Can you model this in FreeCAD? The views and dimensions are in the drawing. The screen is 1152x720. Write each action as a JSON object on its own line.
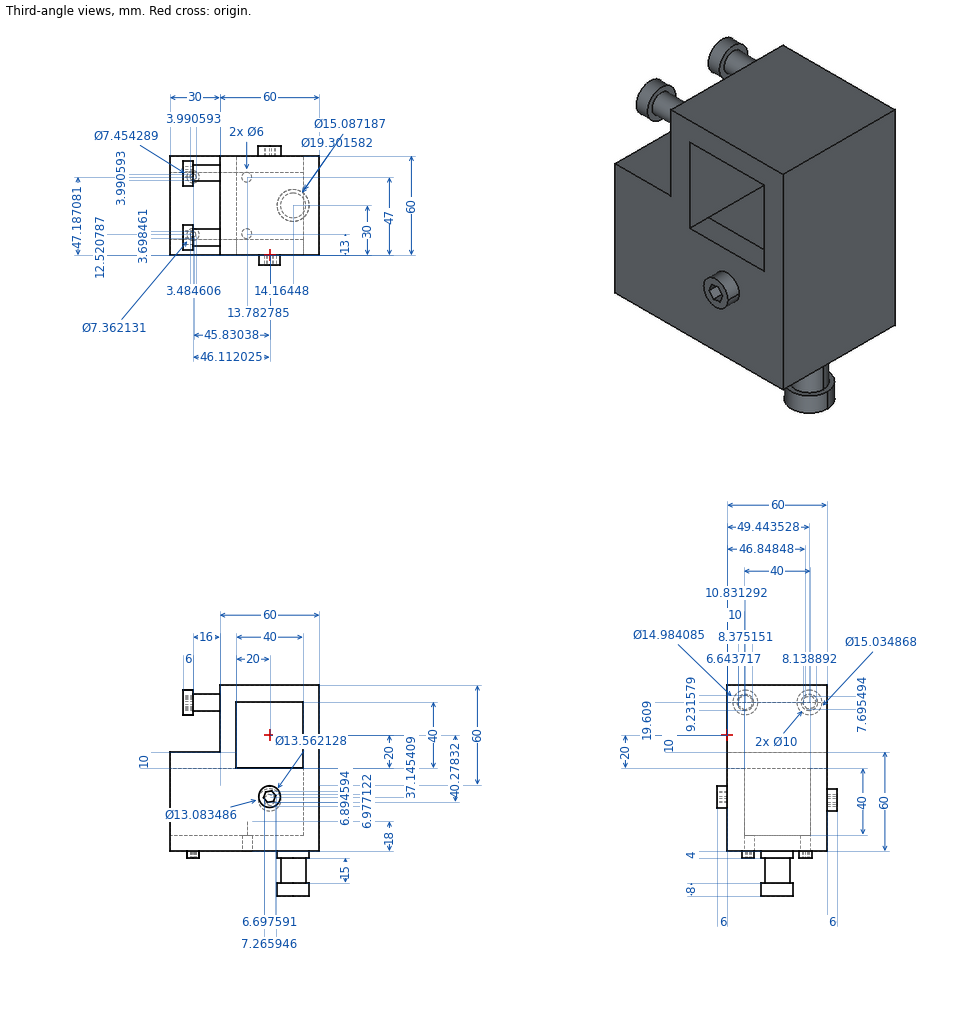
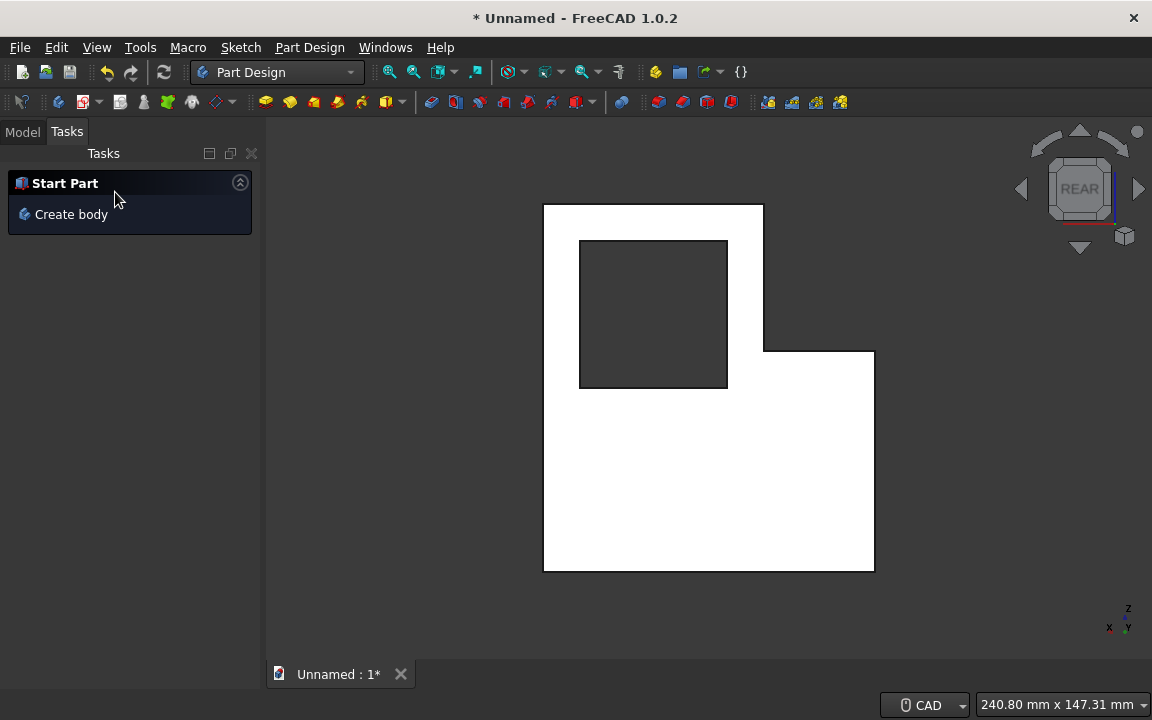
{"action": "key", "text": "5"}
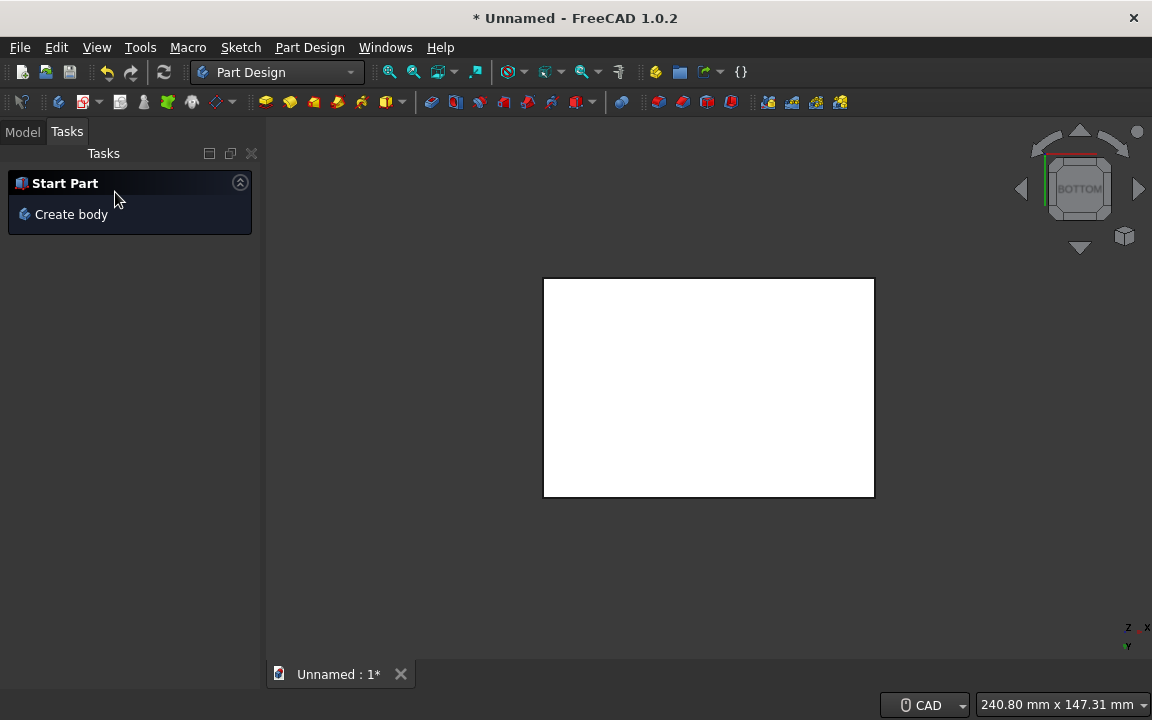
{"action": "left_click", "coordinate": [390, 72]}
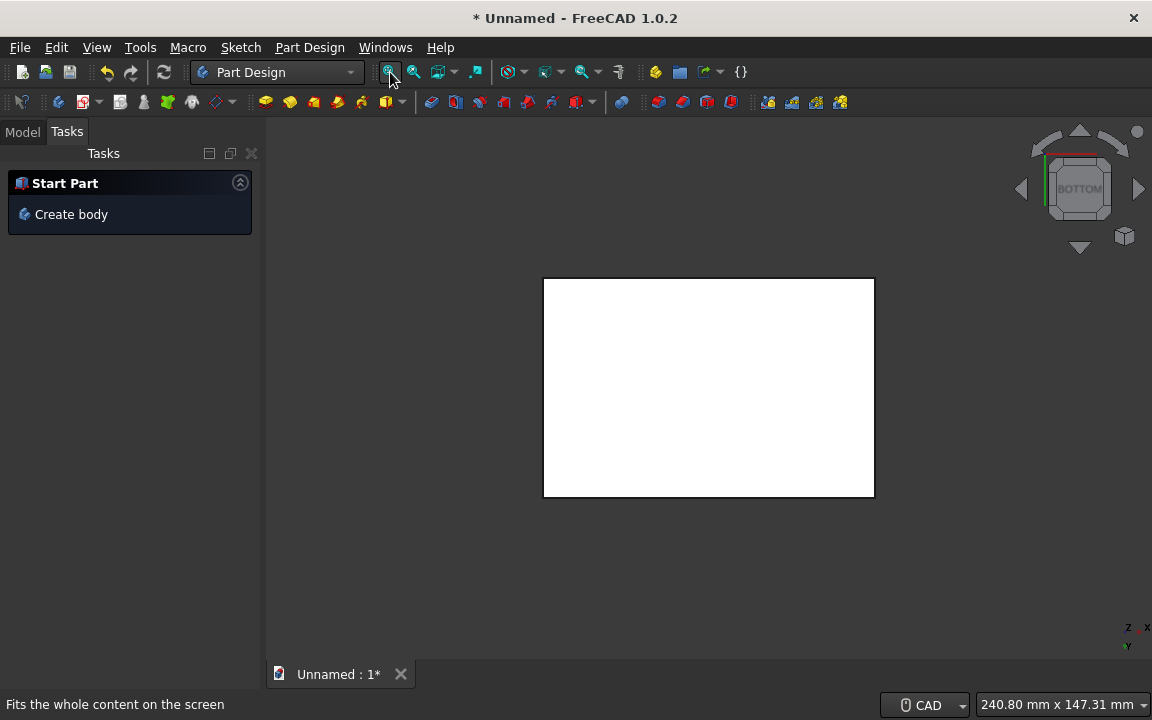
{"action": "left_click", "coordinate": [756, 387]}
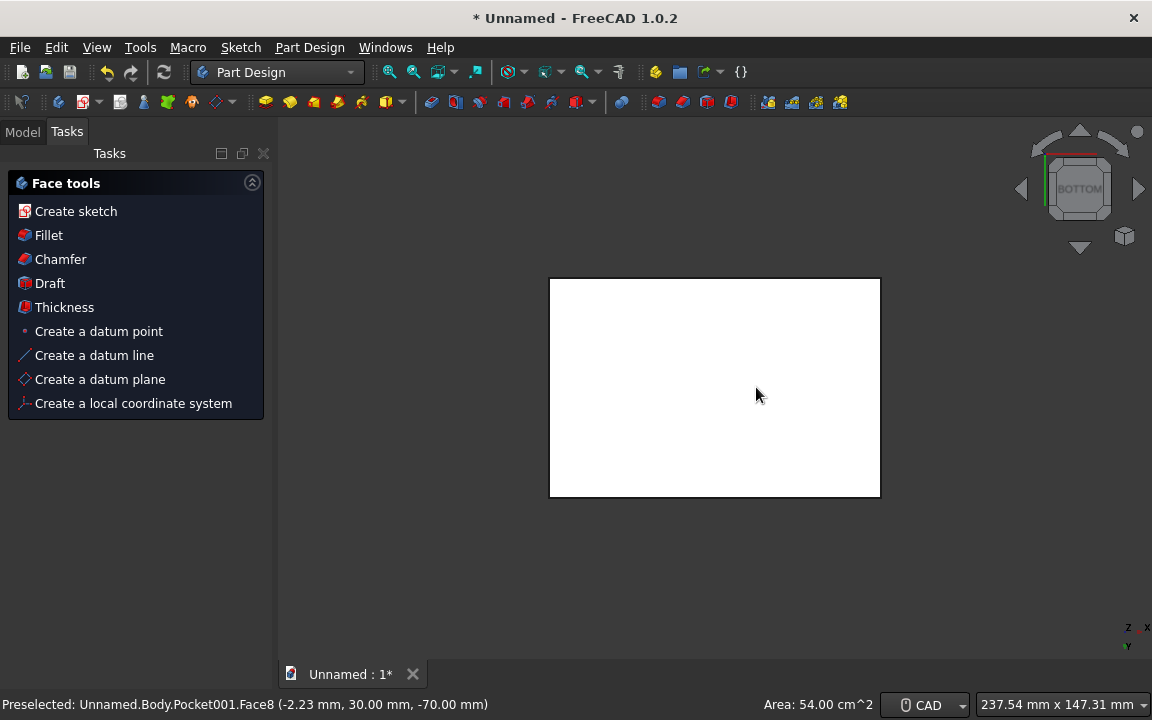
{"action": "left_click", "coordinate": [84, 102]}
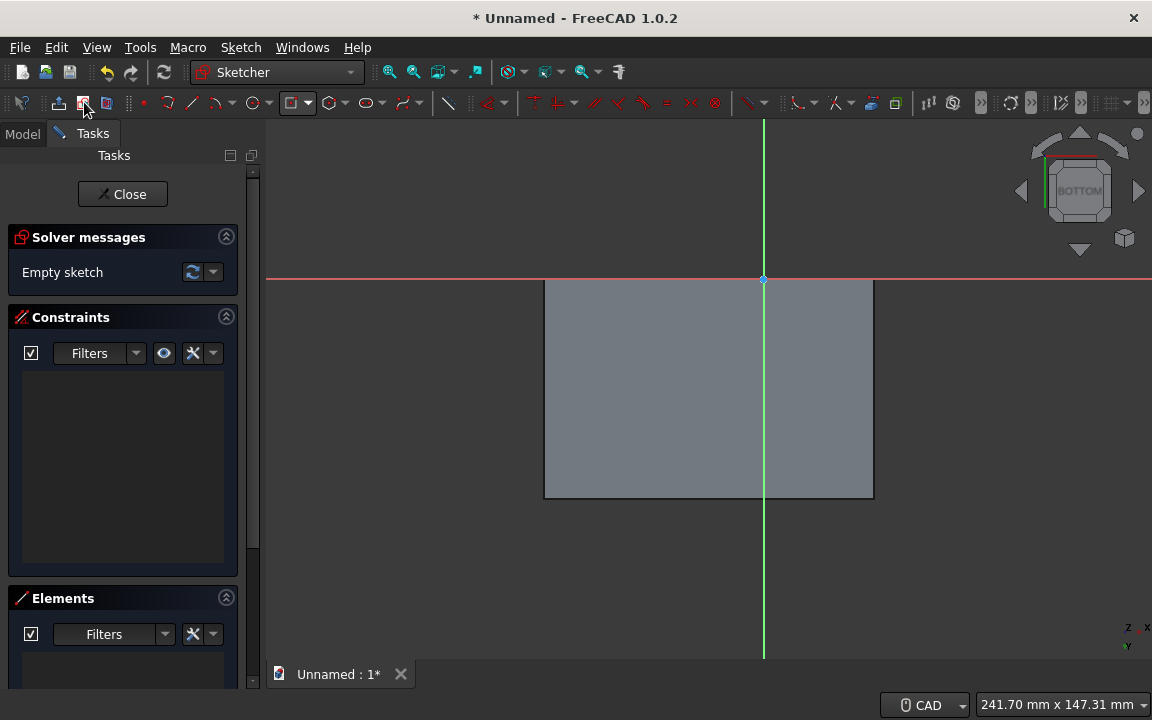
{"action": "scroll", "coordinate": [944, 321], "scroll_direction": "up", "scroll_amount": 4}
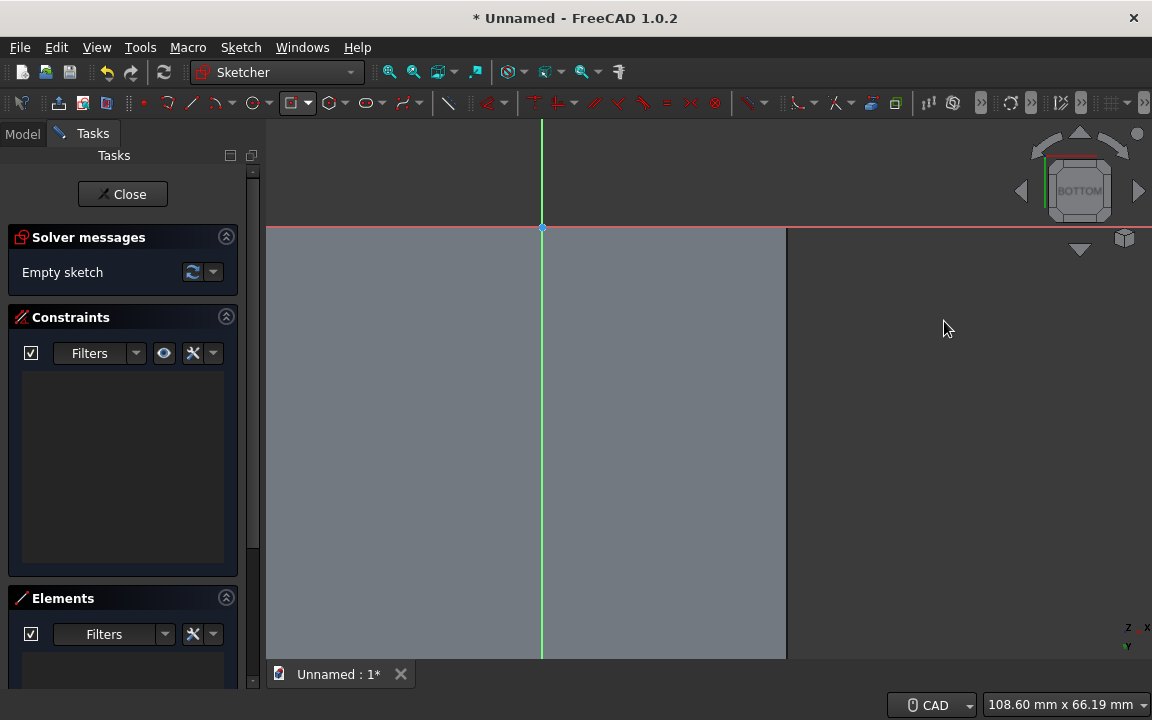
{"action": "left_click", "coordinate": [254, 104]}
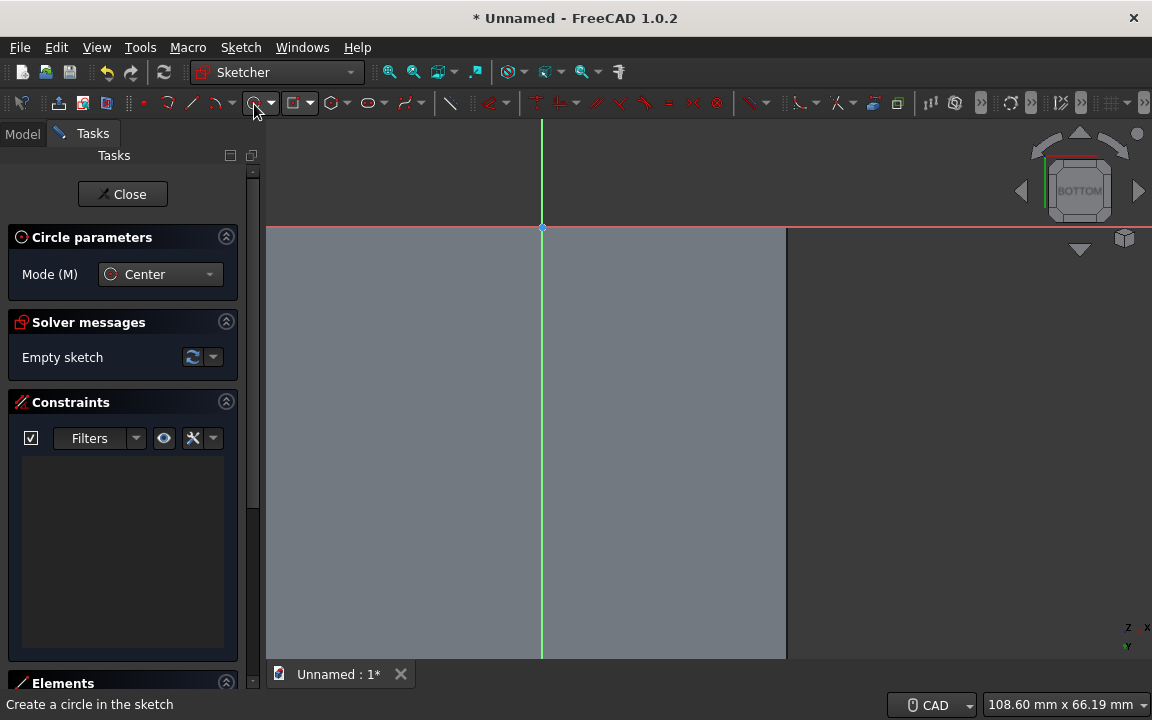
{"action": "left_click", "coordinate": [658, 472]}
{"action": "left_click", "coordinate": [714, 416]}
{"action": "key", "text": "Escape"}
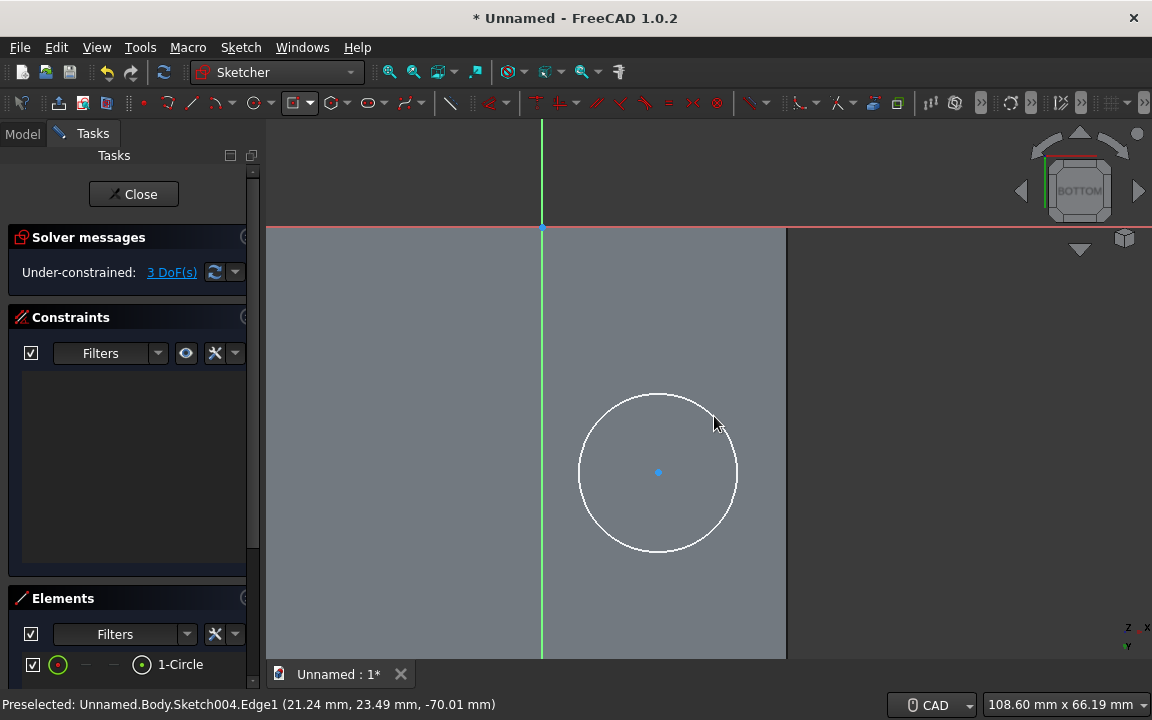
{"action": "left_click", "coordinate": [490, 104]}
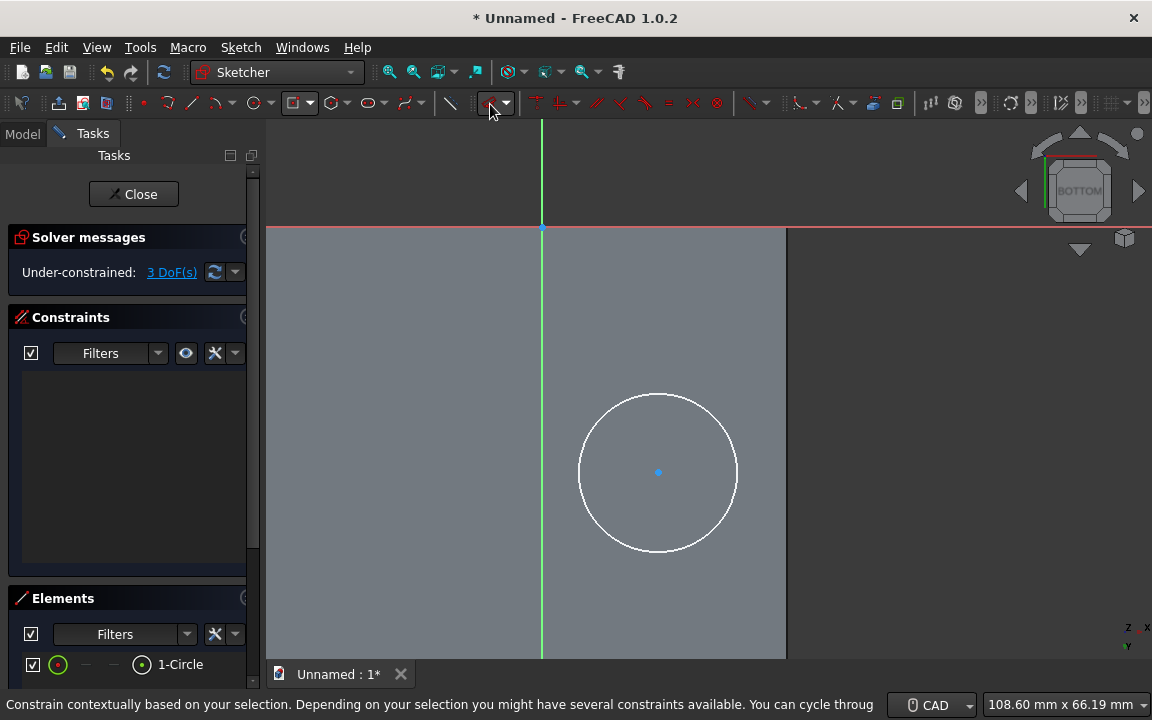
{"action": "left_click", "coordinate": [714, 417]}
{"action": "left_click", "coordinate": [737, 394]}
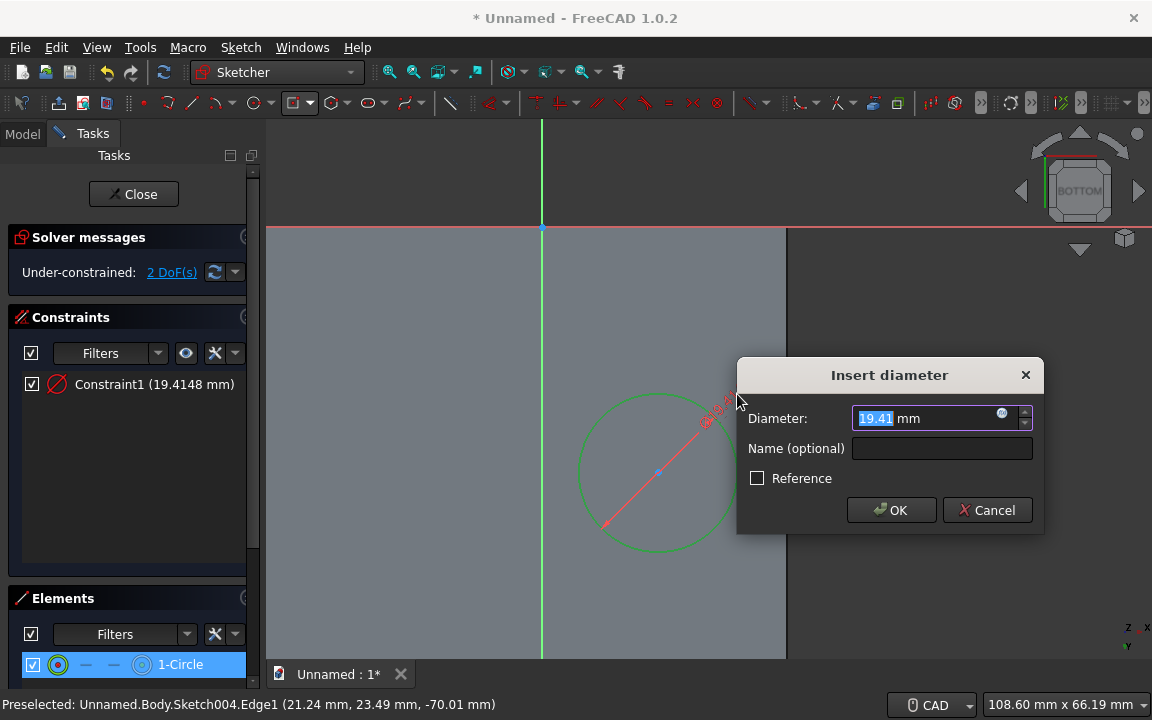
{"action": "type", "text": "19.301582"}
{"action": "key", "text": "Return"}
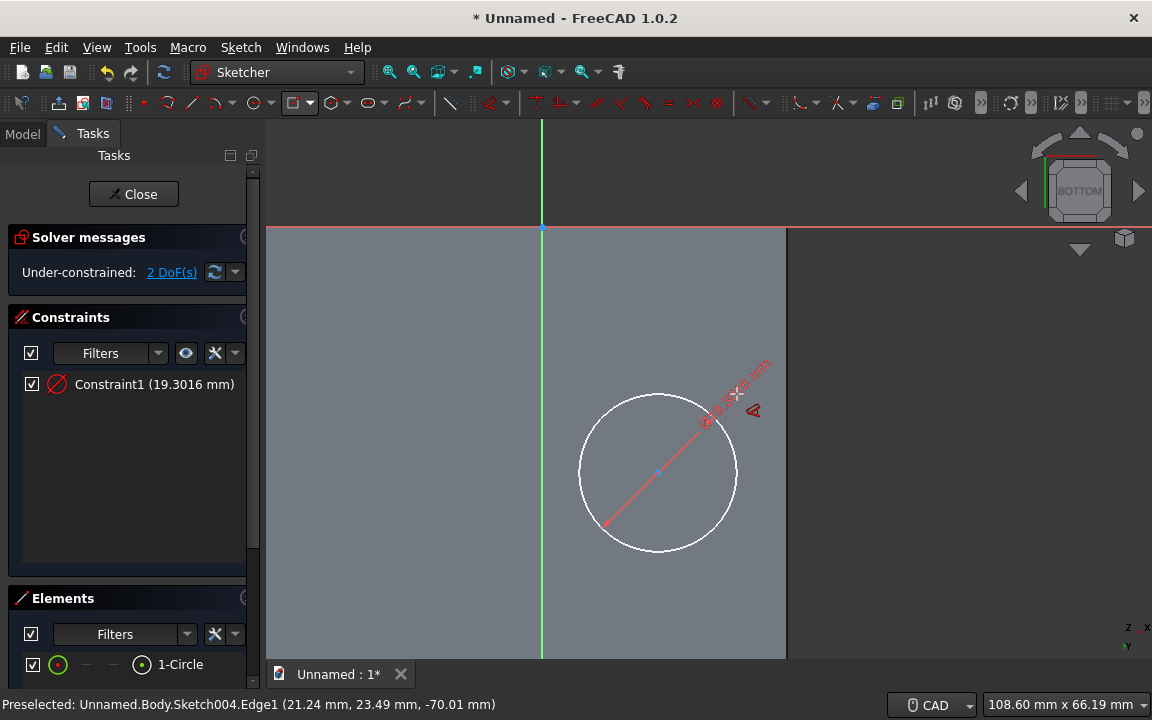
{"action": "left_click", "coordinate": [658, 473]}
{"action": "left_click", "coordinate": [508, 350]}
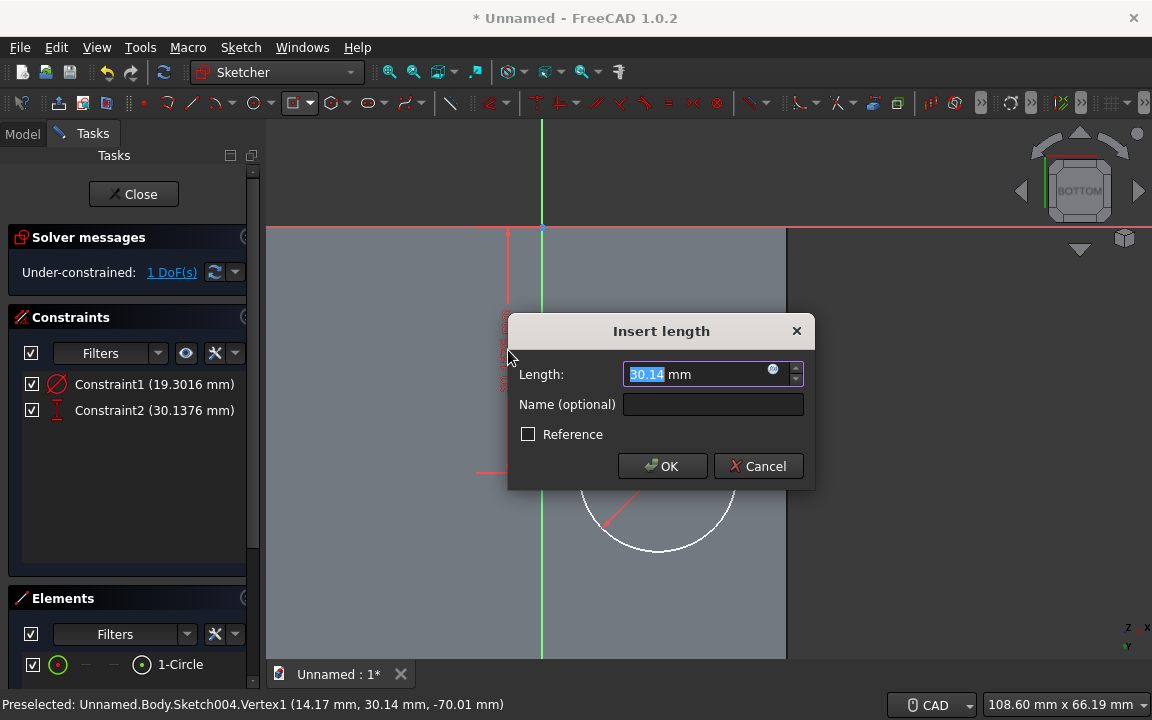
{"action": "type", "text": "30"}
{"action": "key", "text": "Return"}